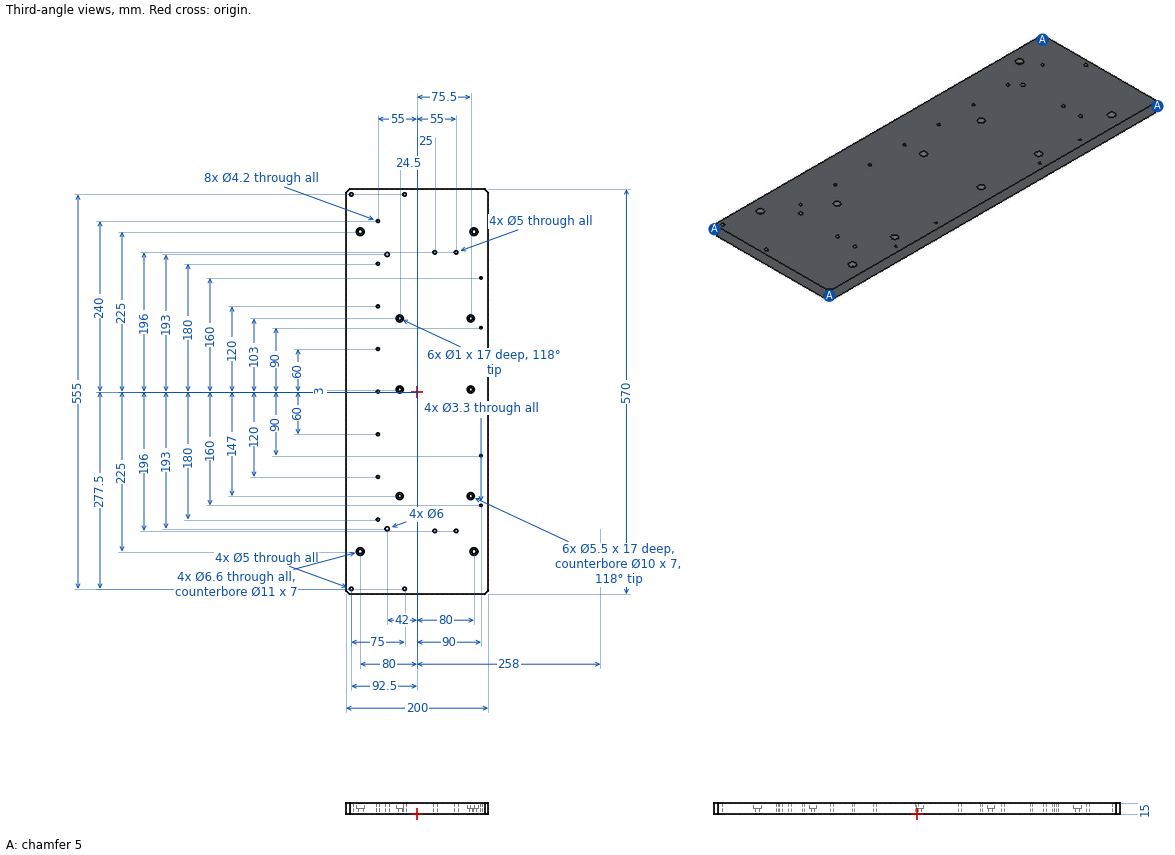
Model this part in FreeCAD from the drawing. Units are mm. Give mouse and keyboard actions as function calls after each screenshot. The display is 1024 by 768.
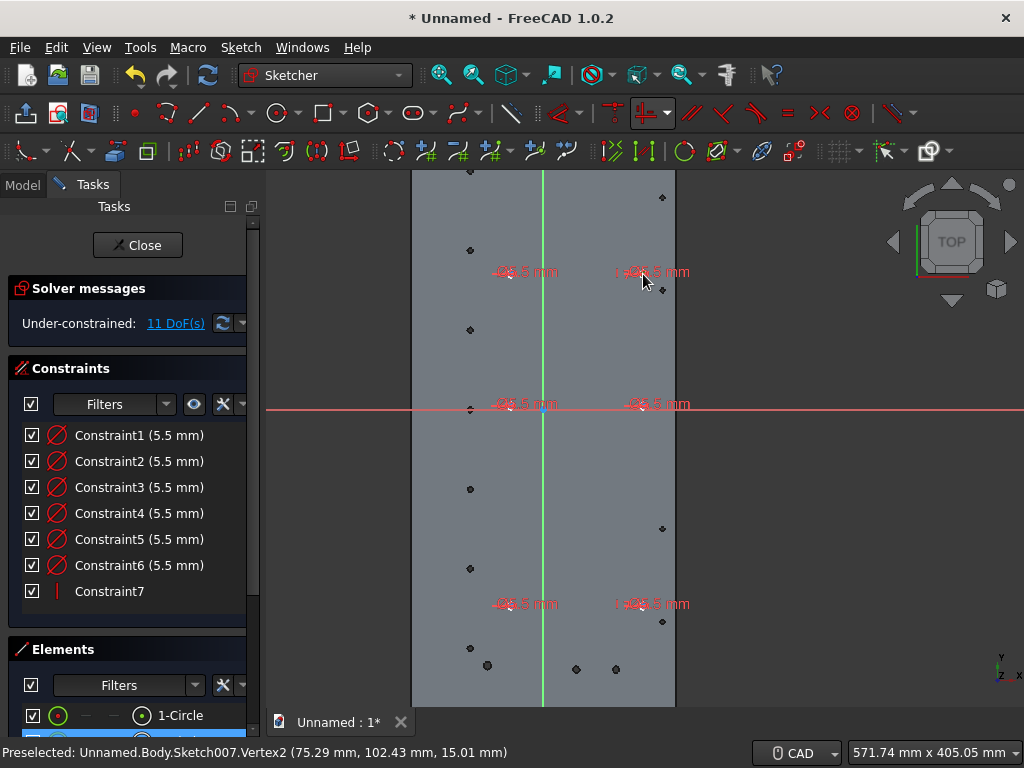
click(643, 406)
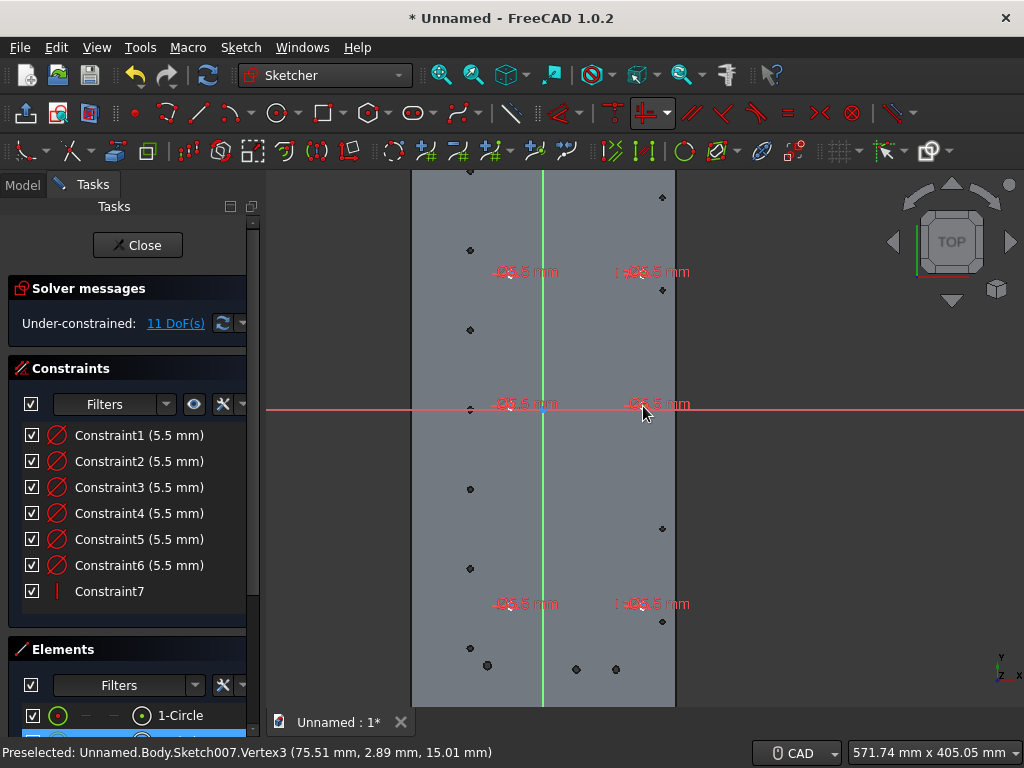
key(v)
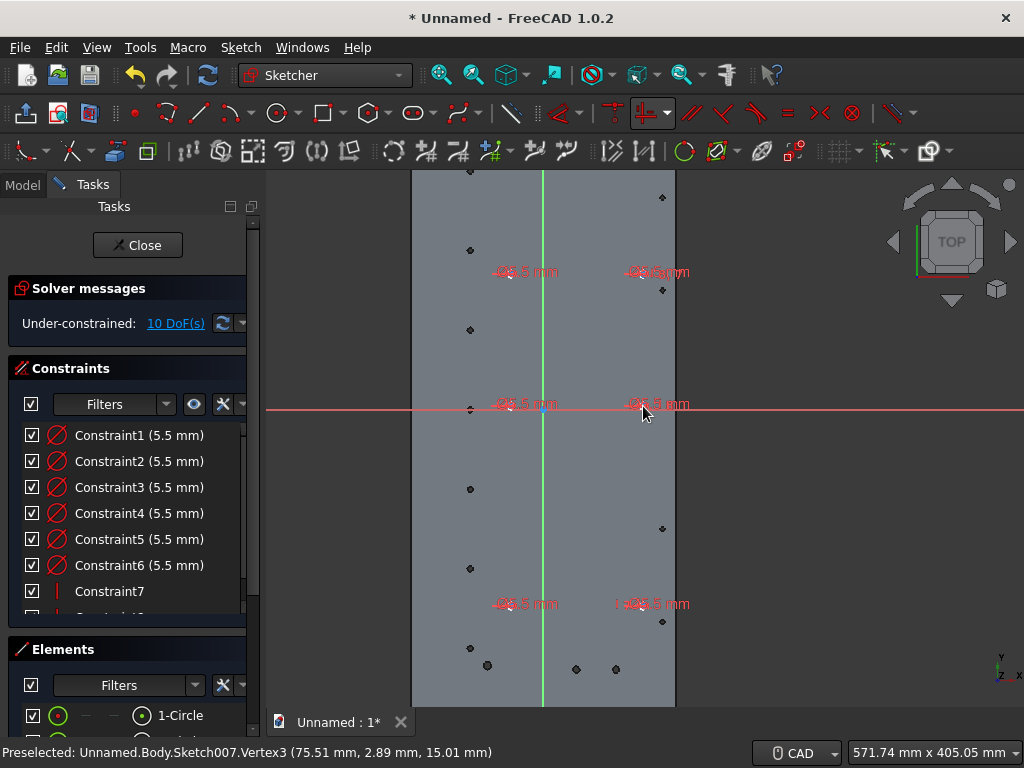
click(643, 274)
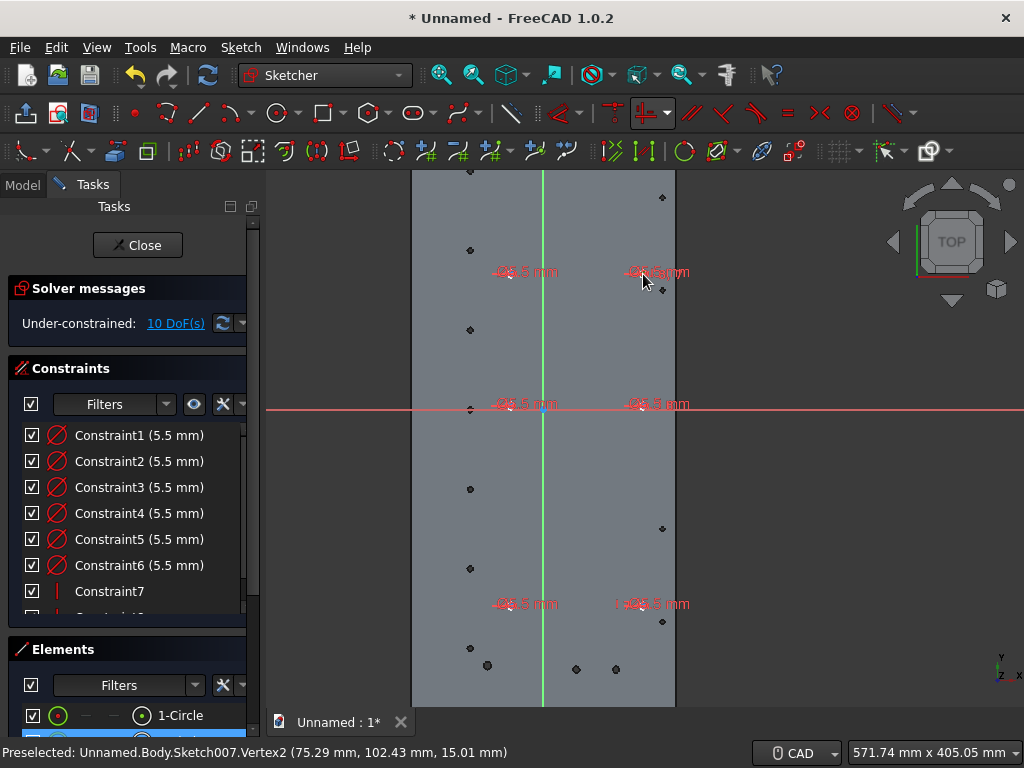
click(511, 274)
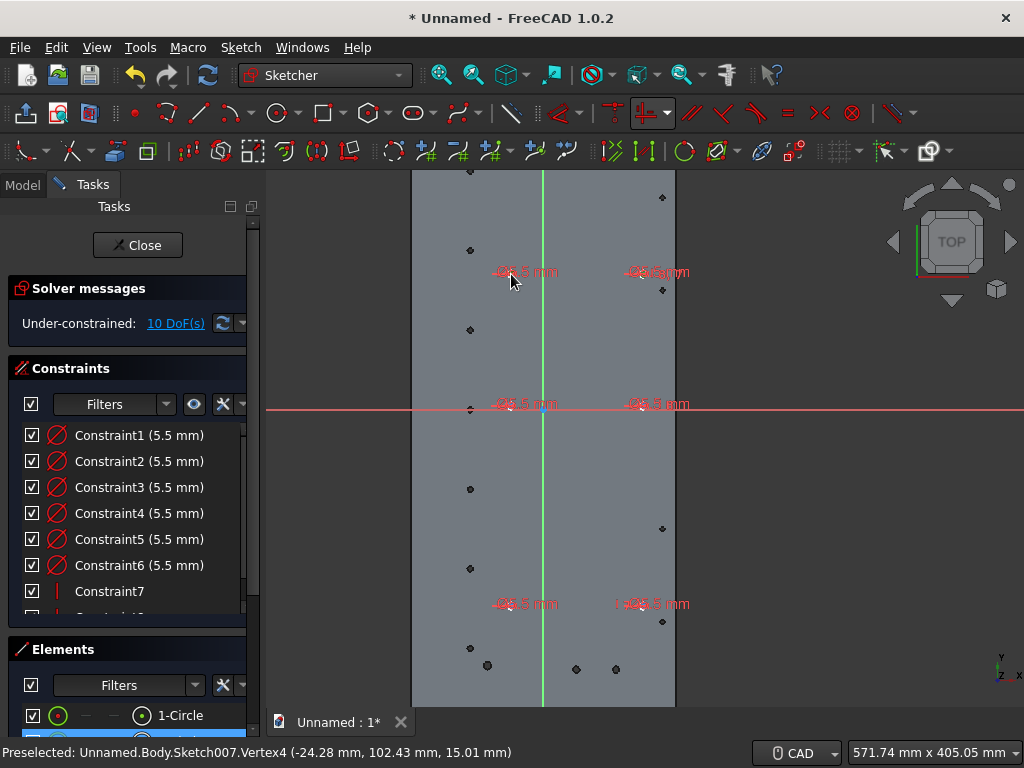
key(h)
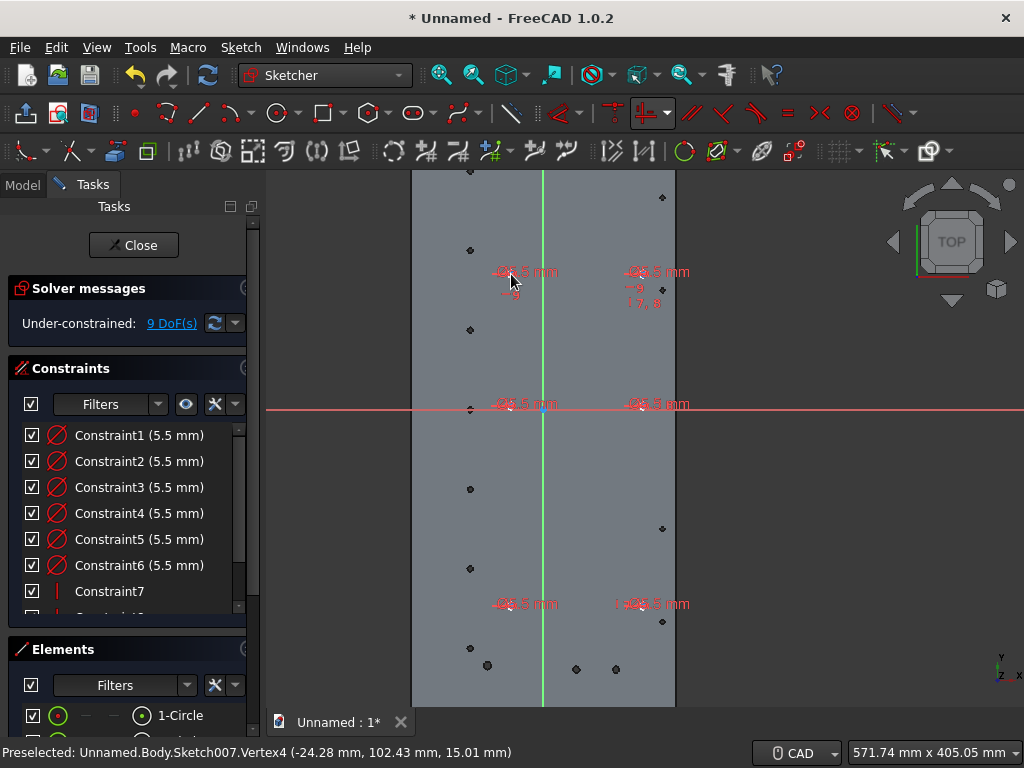
click(511, 274)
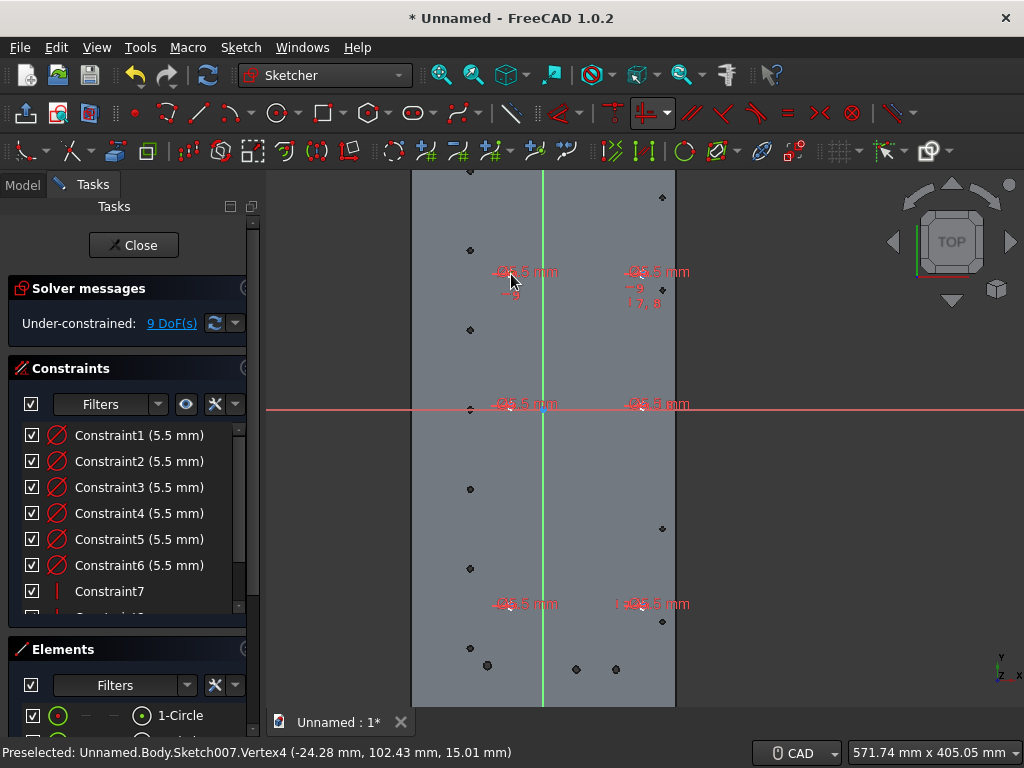
click(511, 406)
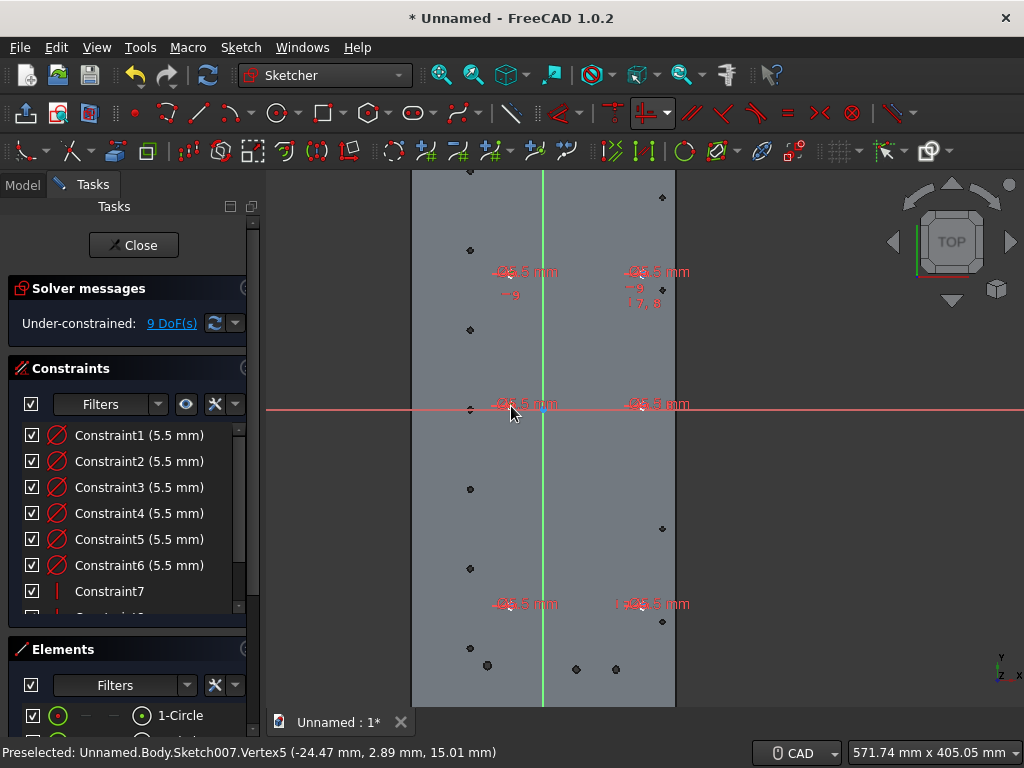
key(v)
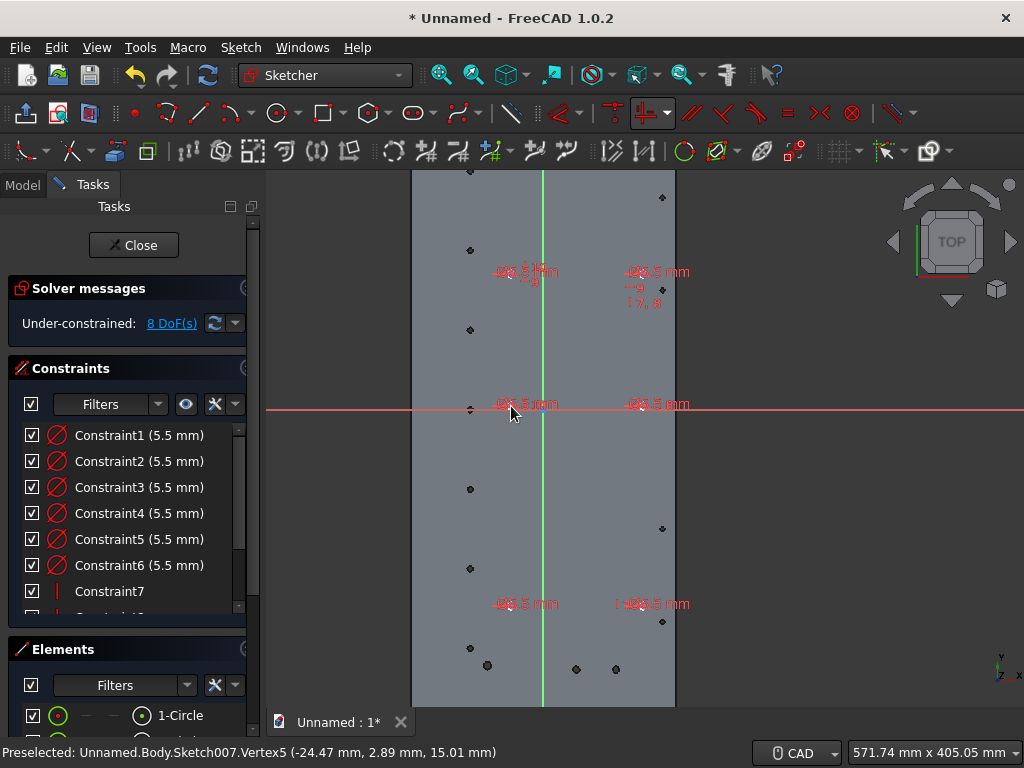
click(643, 406)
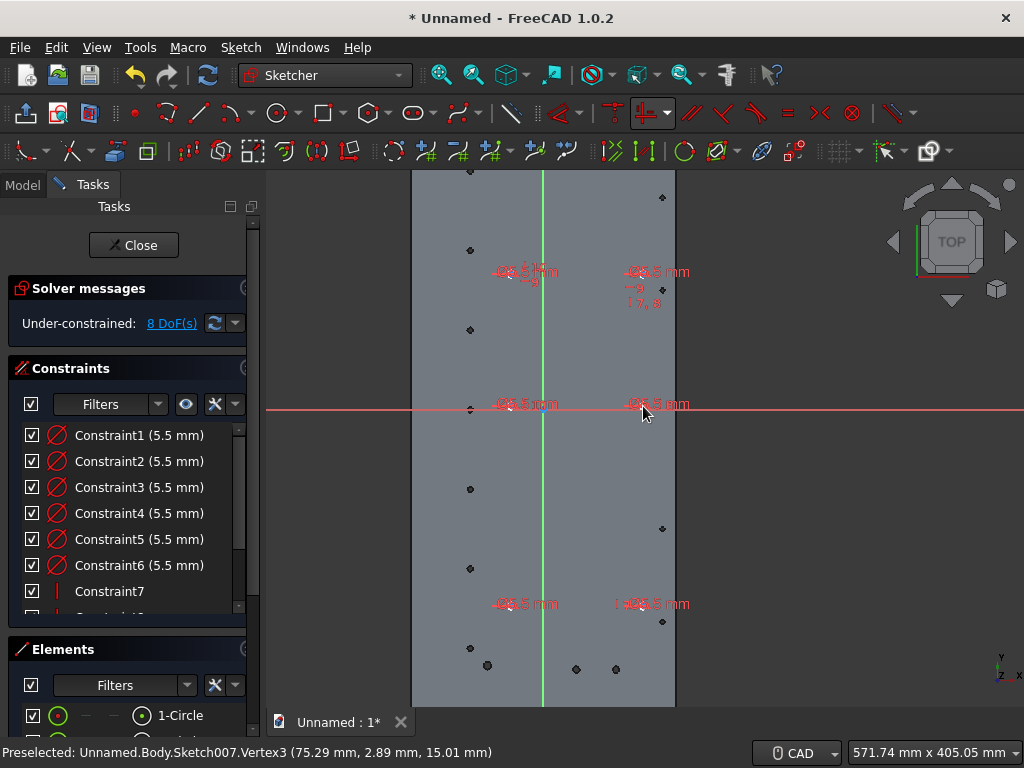
click(511, 406)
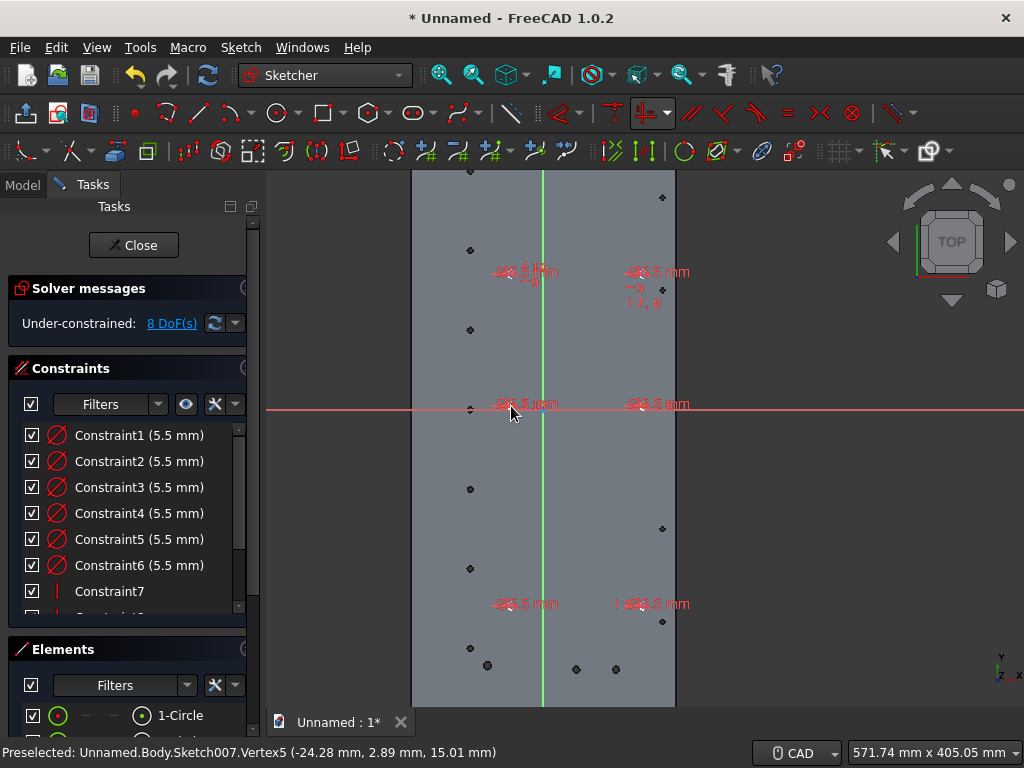
click(670, 114)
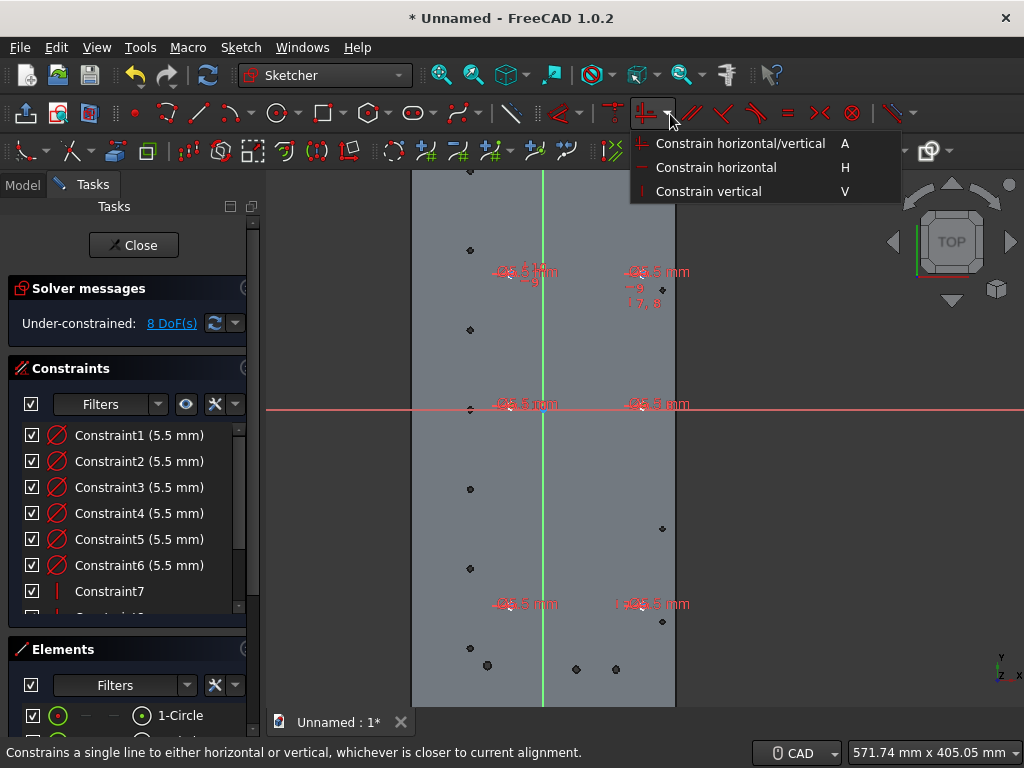
click(766, 167)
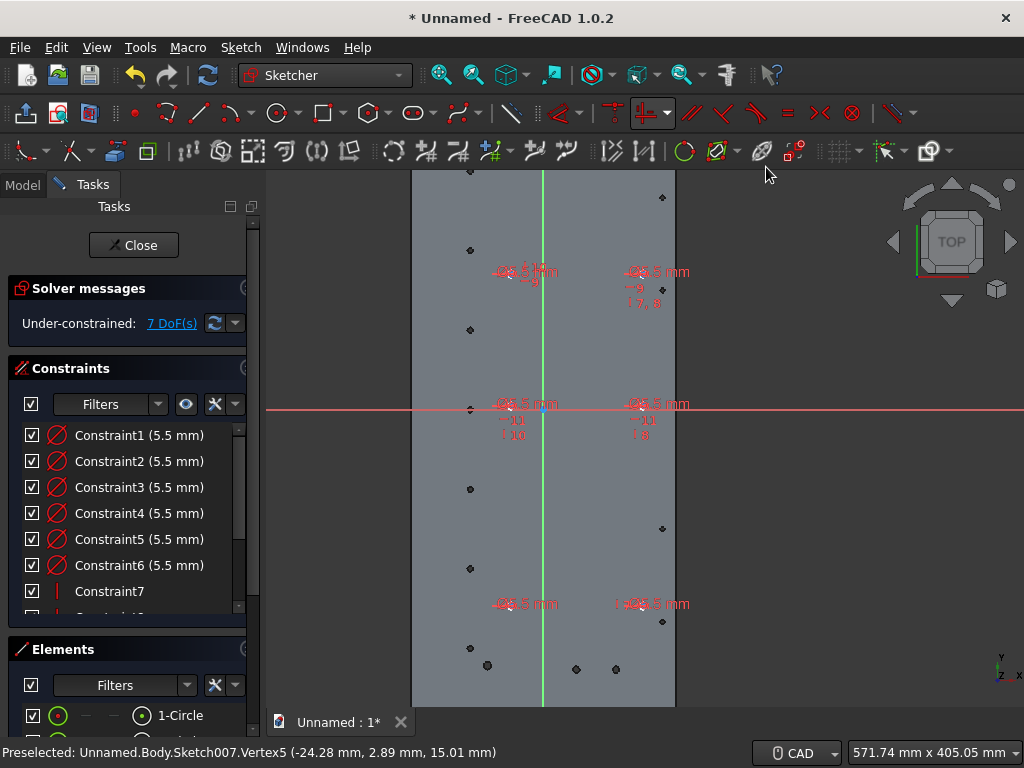
click(511, 406)